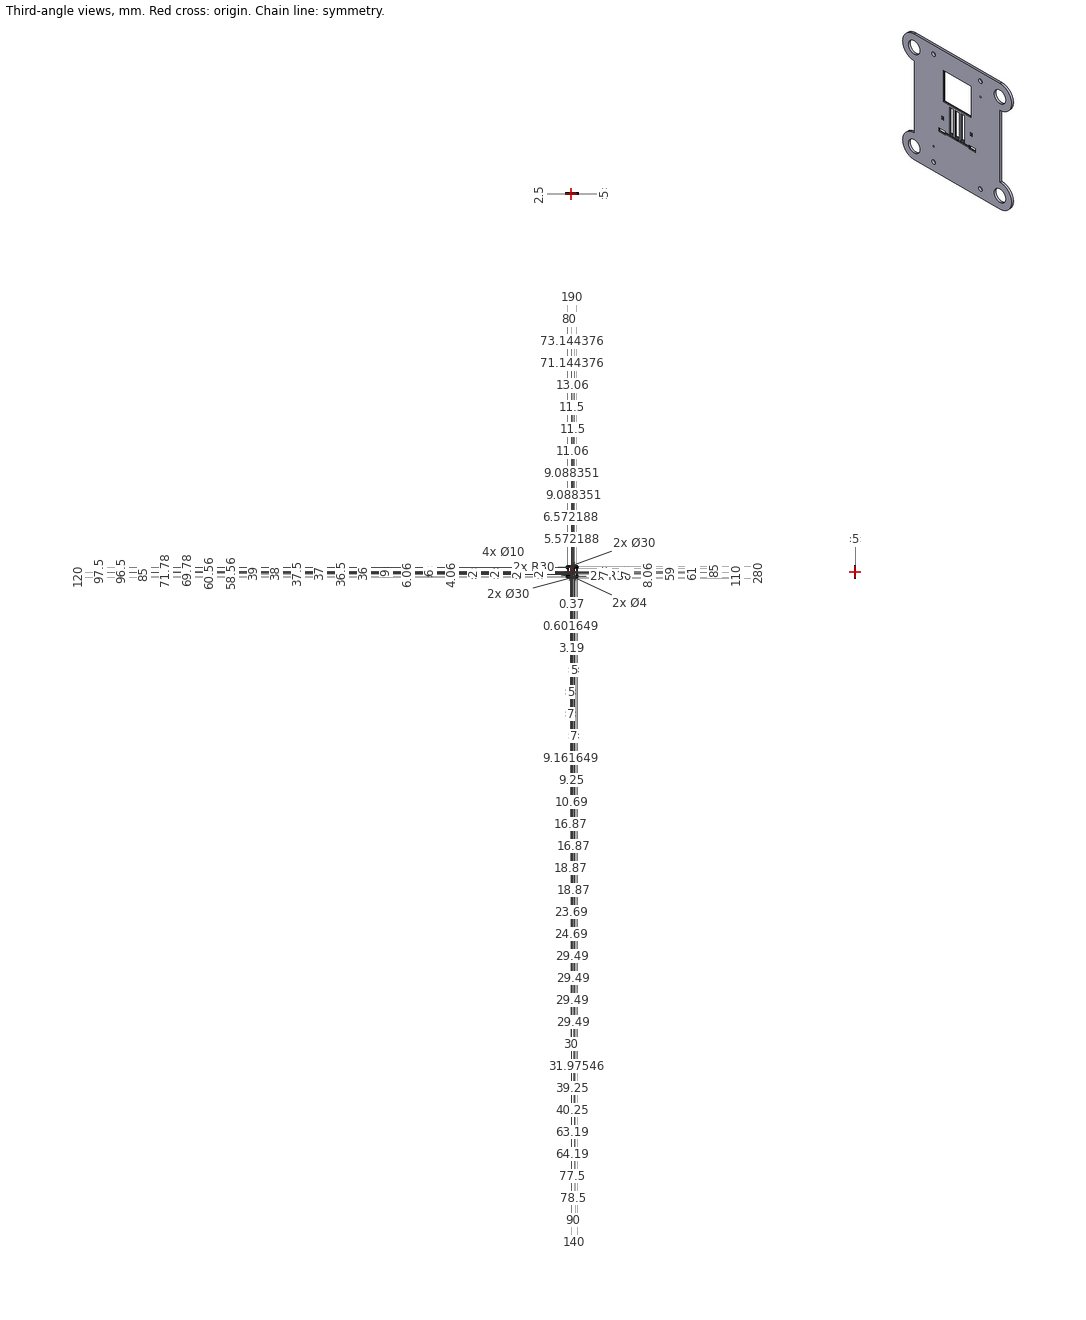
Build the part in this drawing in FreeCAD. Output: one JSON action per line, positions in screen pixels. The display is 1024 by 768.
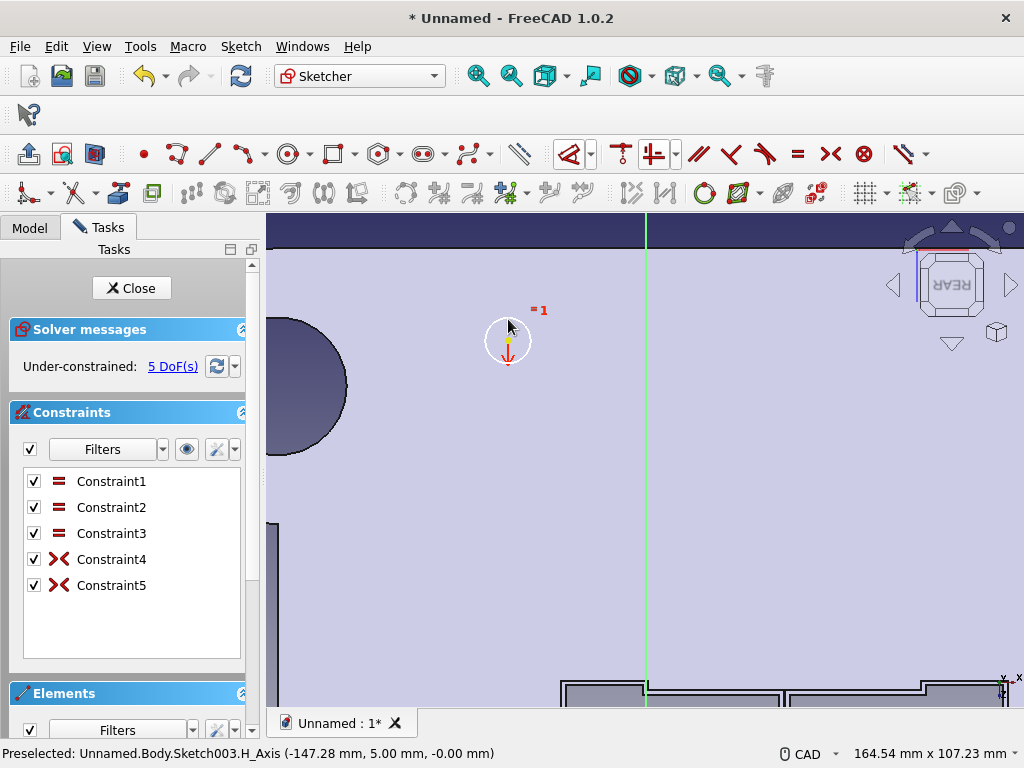
{"action": "left_click", "coordinate": [509, 318]}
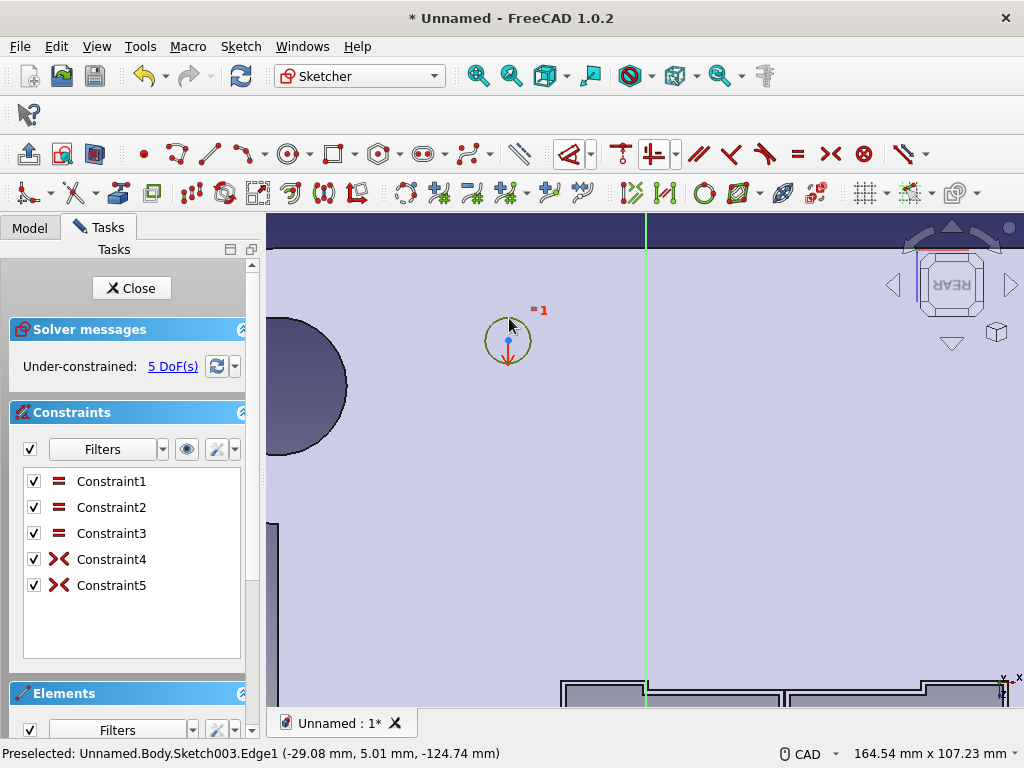
{"action": "left_click", "coordinate": [590, 154]}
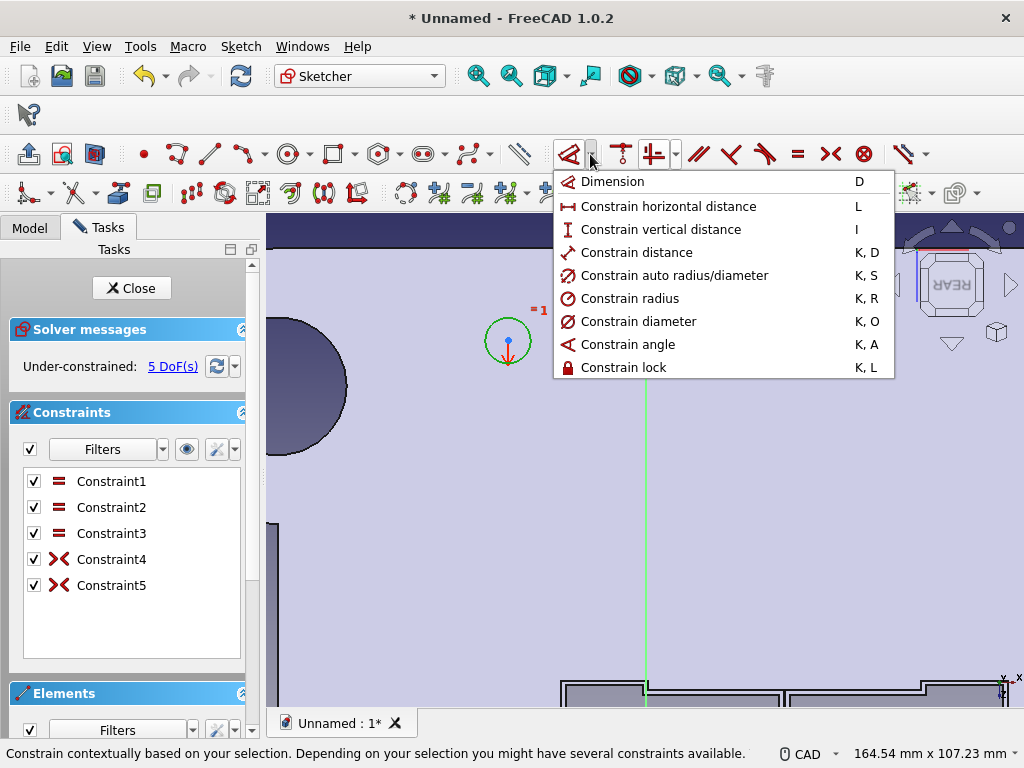
{"action": "left_click", "coordinate": [724, 322]}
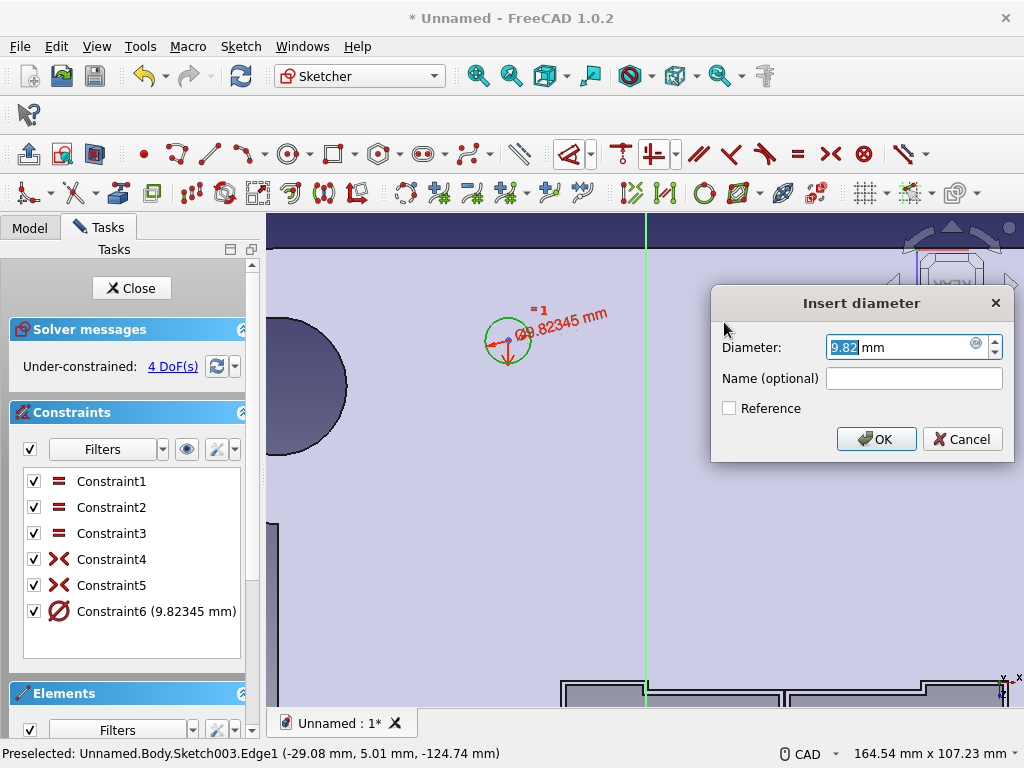
{"action": "type", "text": "10"}
{"action": "key", "text": "Return"}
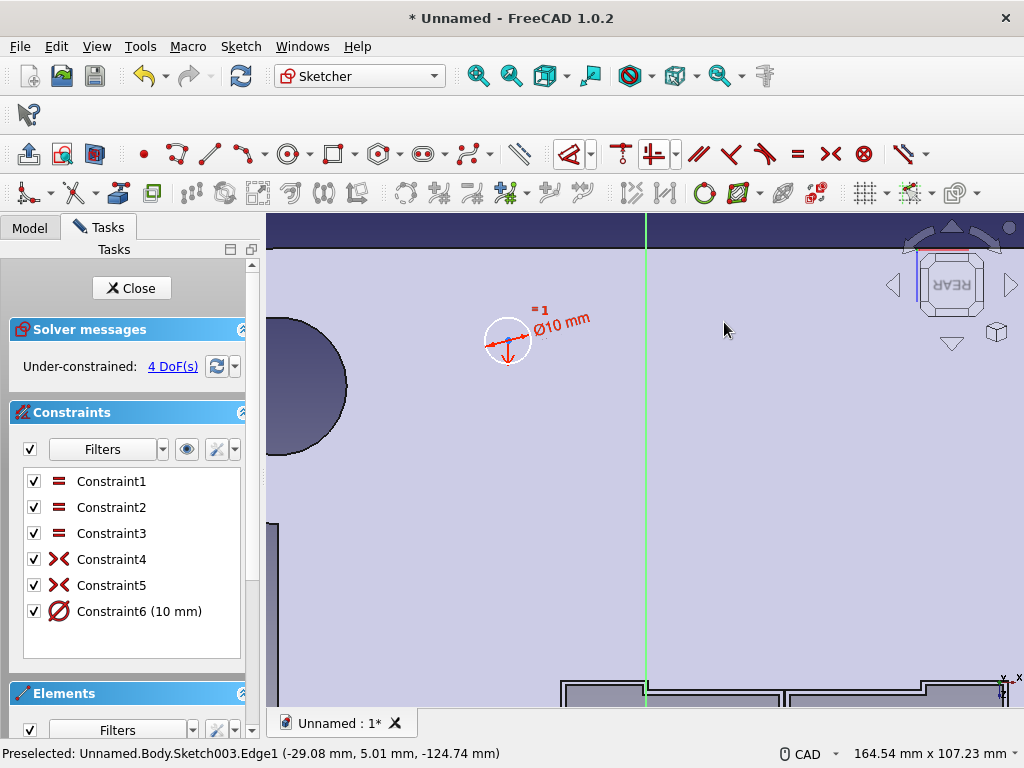
{"action": "left_click", "coordinate": [508, 341]}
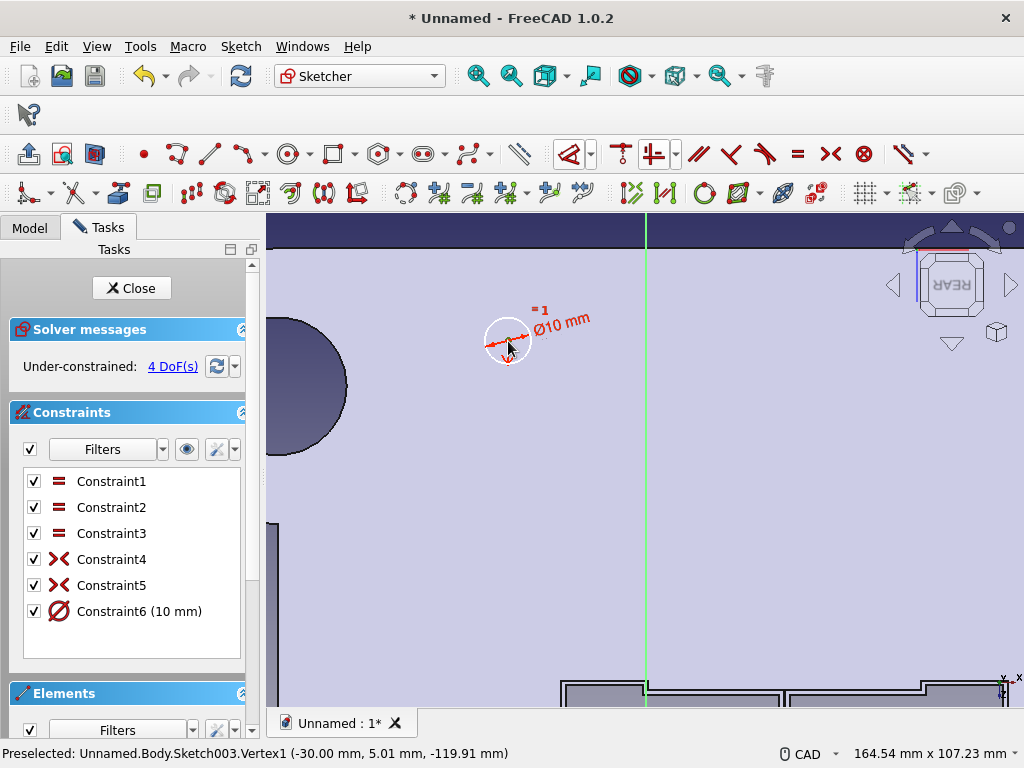
{"action": "left_click", "coordinate": [590, 154]}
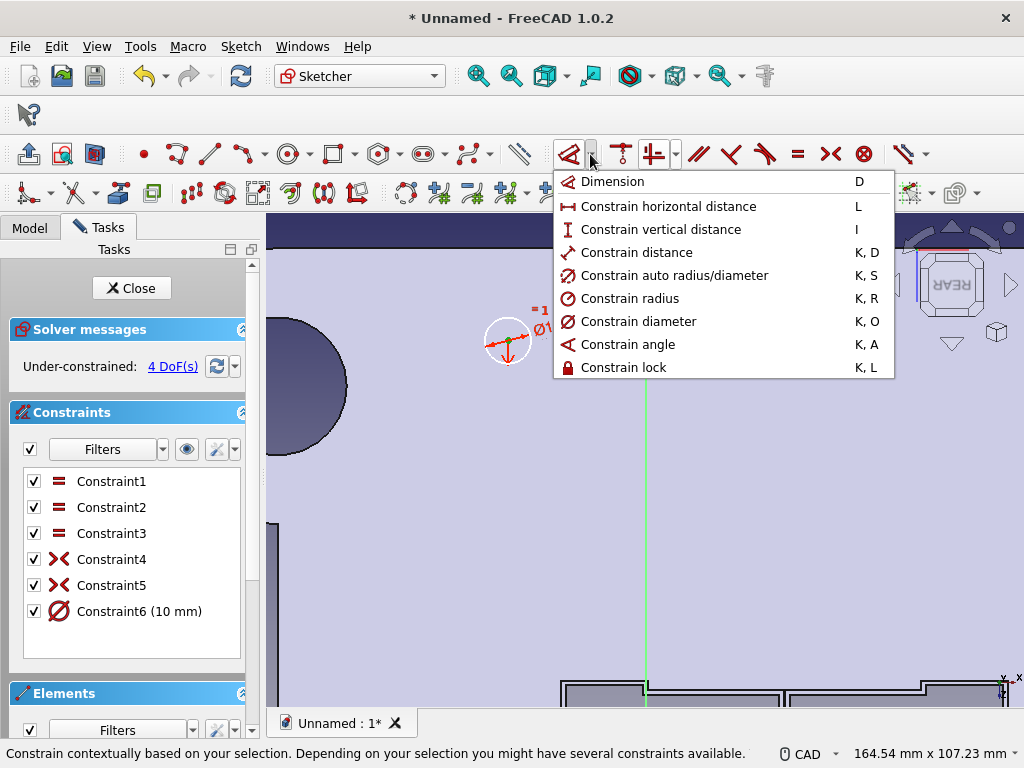
{"action": "left_click", "coordinate": [724, 206]}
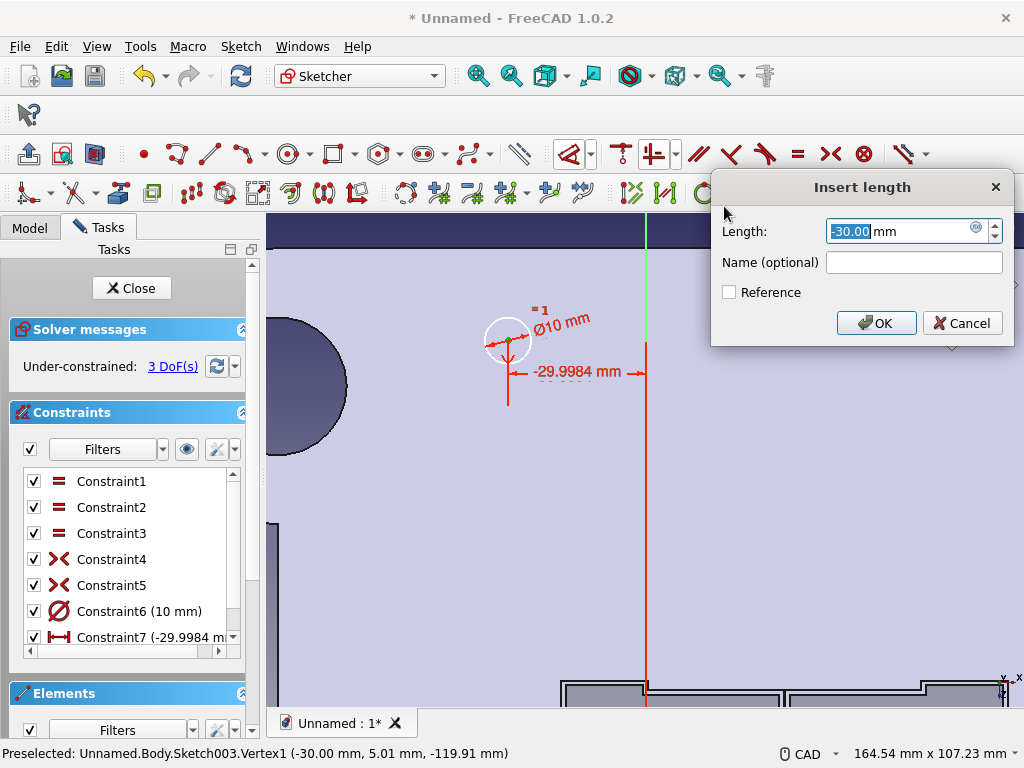
{"action": "type", "text": "-30"}
{"action": "key", "text": "Return"}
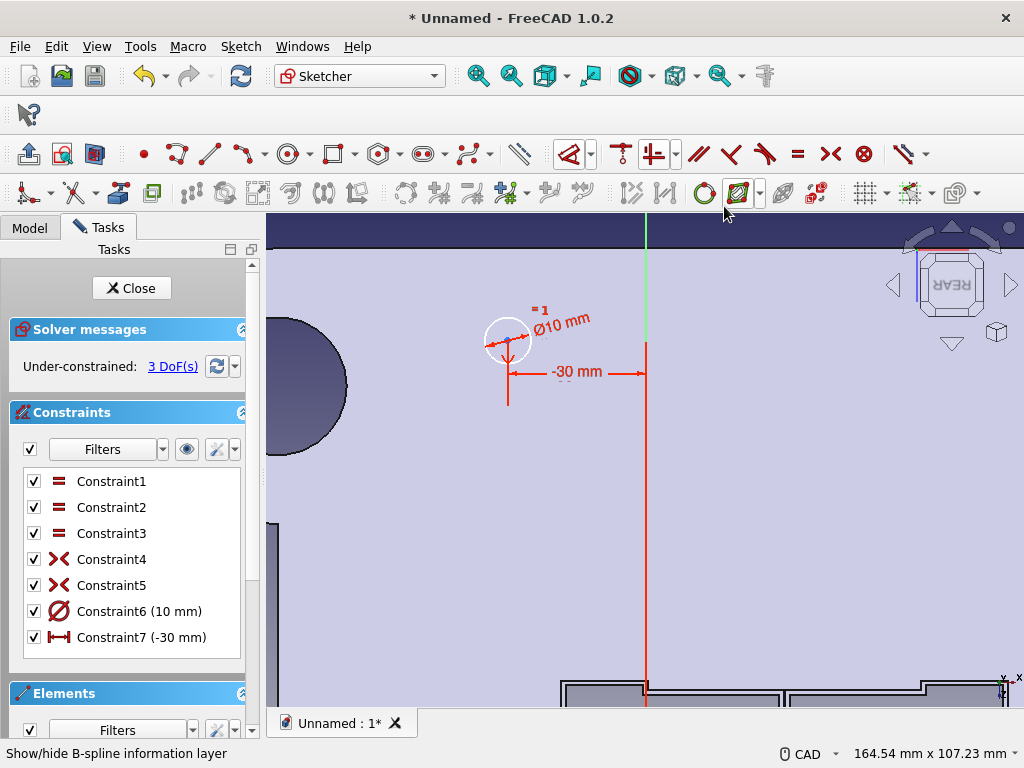
{"action": "scroll", "coordinate": [508, 318], "scroll_direction": "down", "scroll_amount": 7}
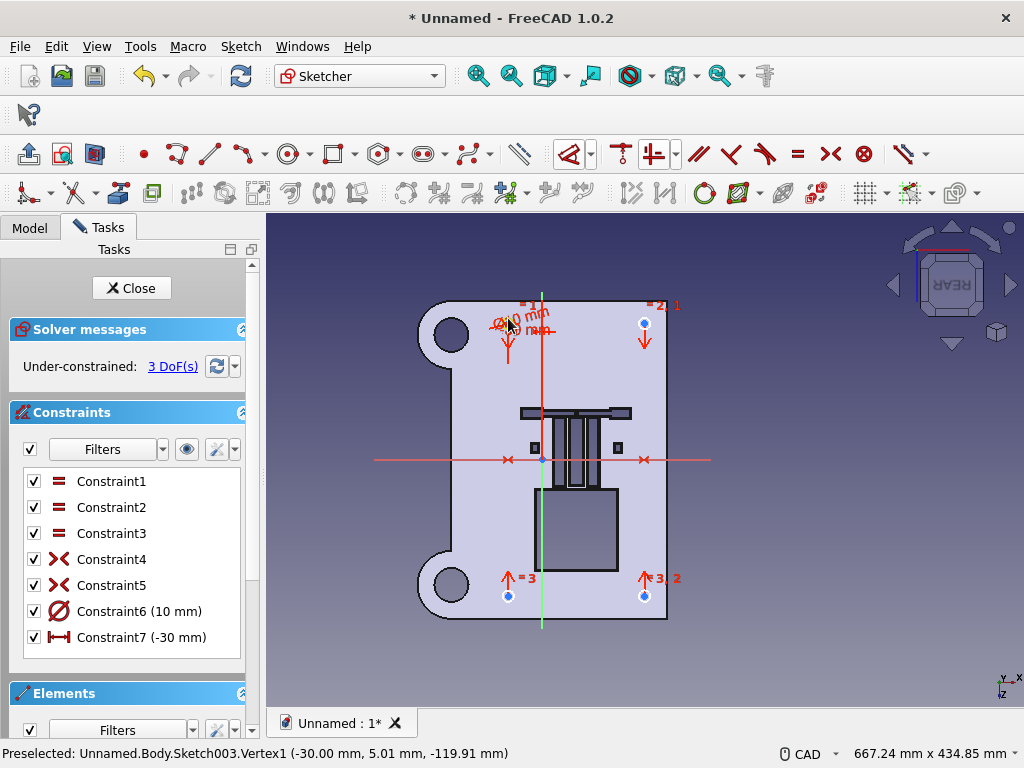
{"action": "left_click", "coordinate": [645, 324]}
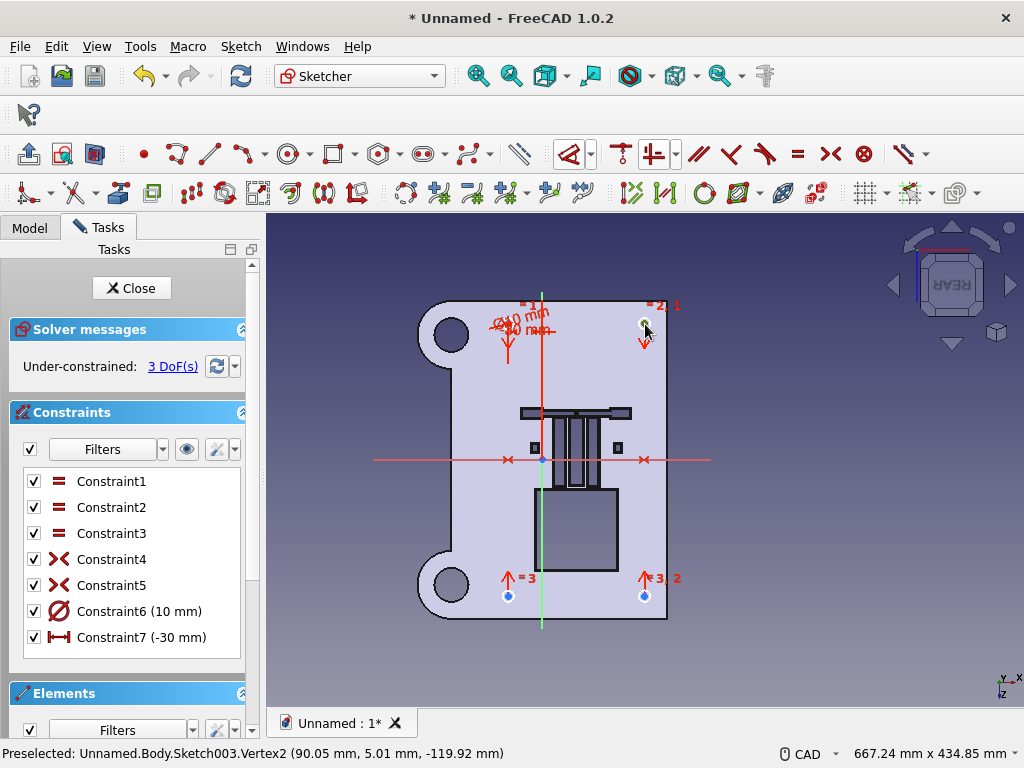
{"action": "key", "text": "l"}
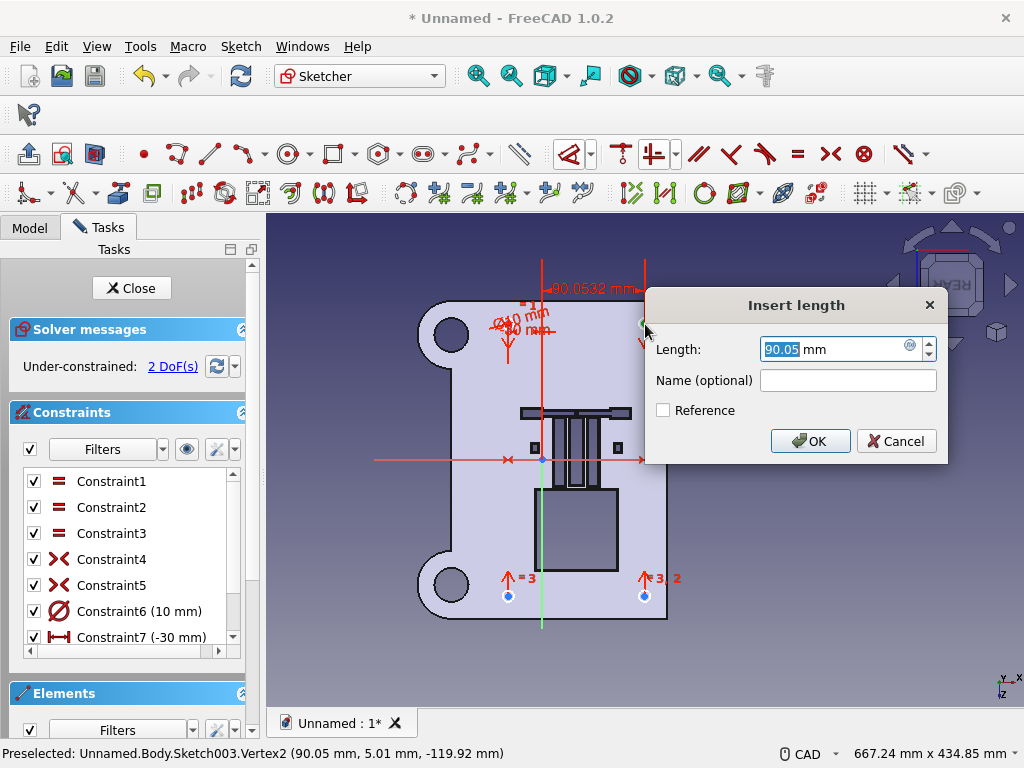
{"action": "type", "text": "90"}
{"action": "key", "text": "Return"}